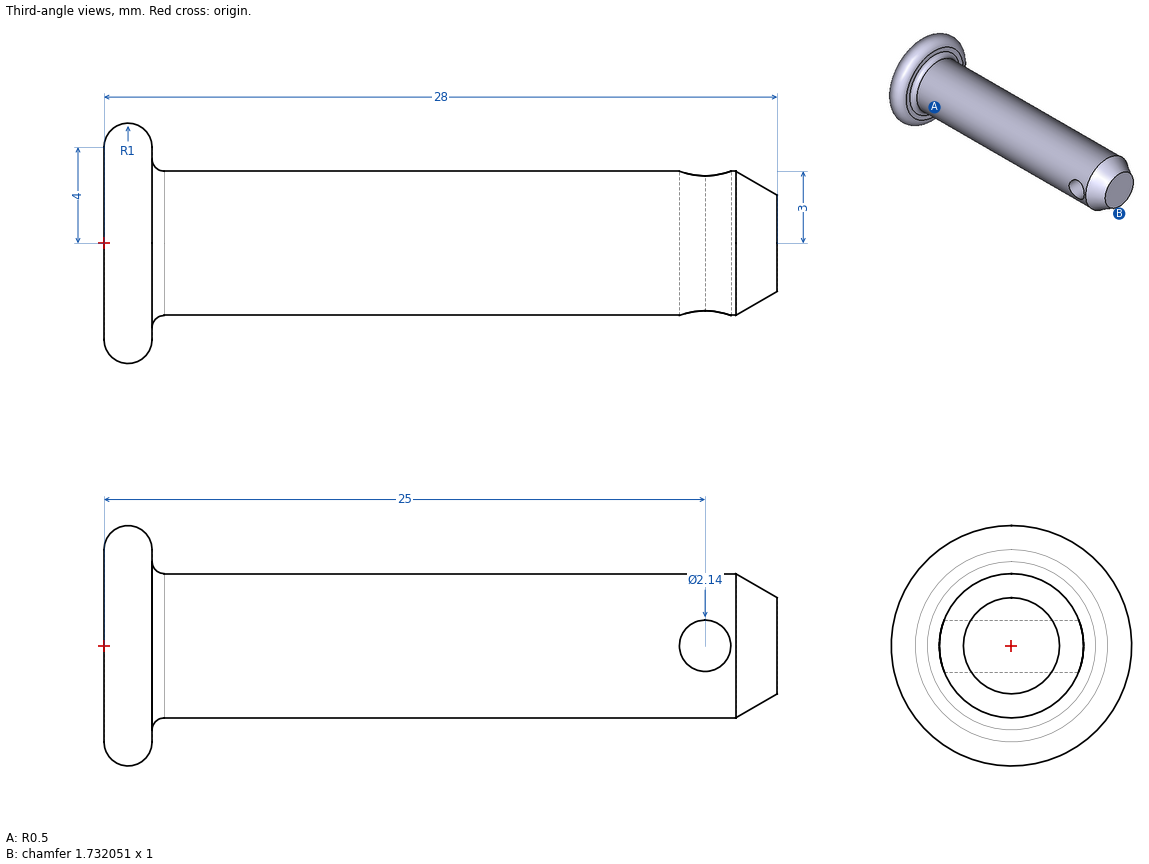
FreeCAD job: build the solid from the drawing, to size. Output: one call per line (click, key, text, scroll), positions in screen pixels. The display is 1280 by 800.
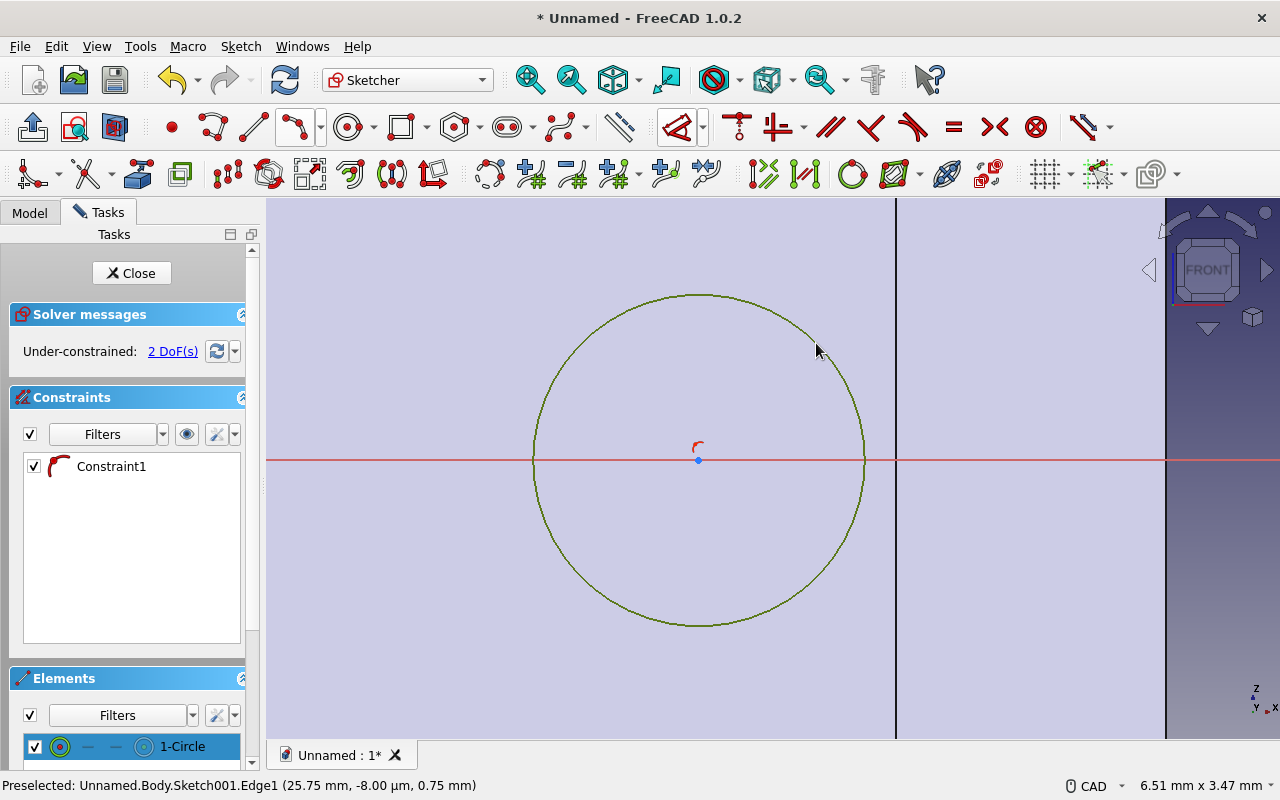
click(702, 128)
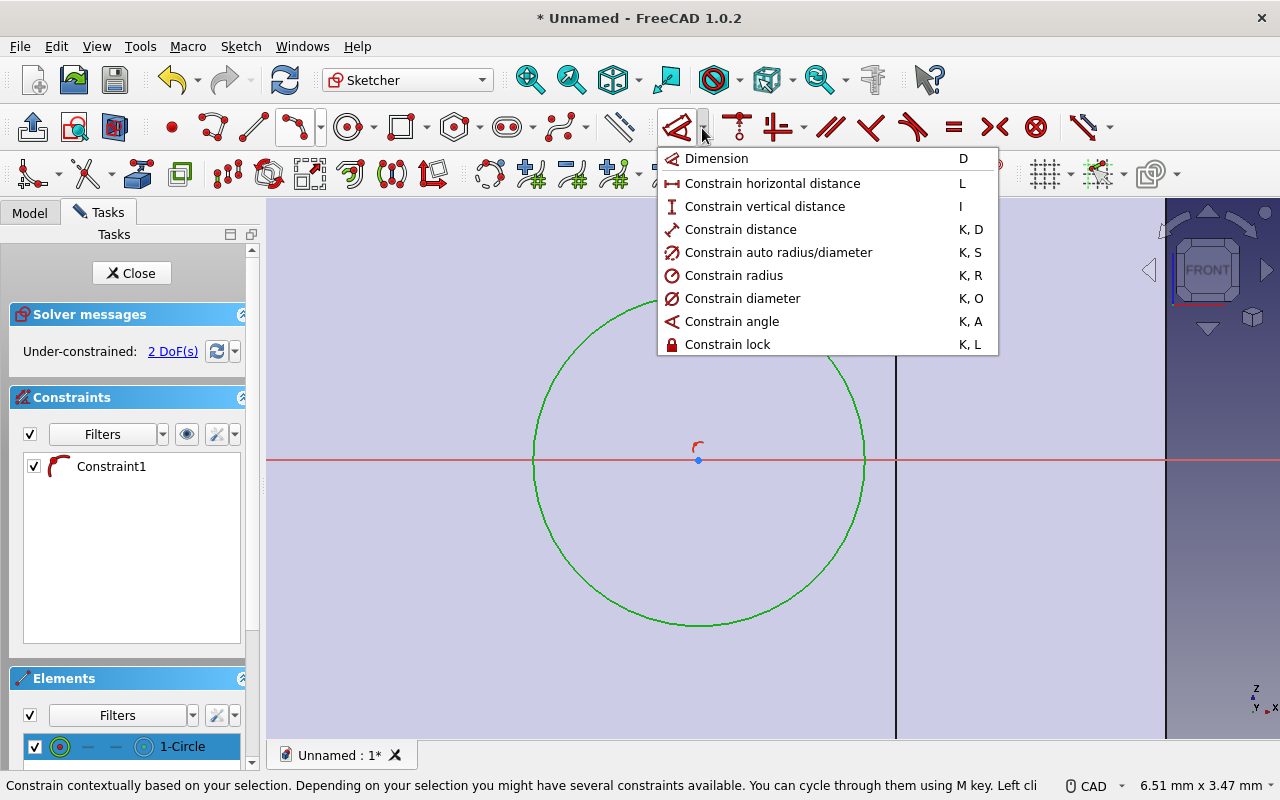
click(828, 298)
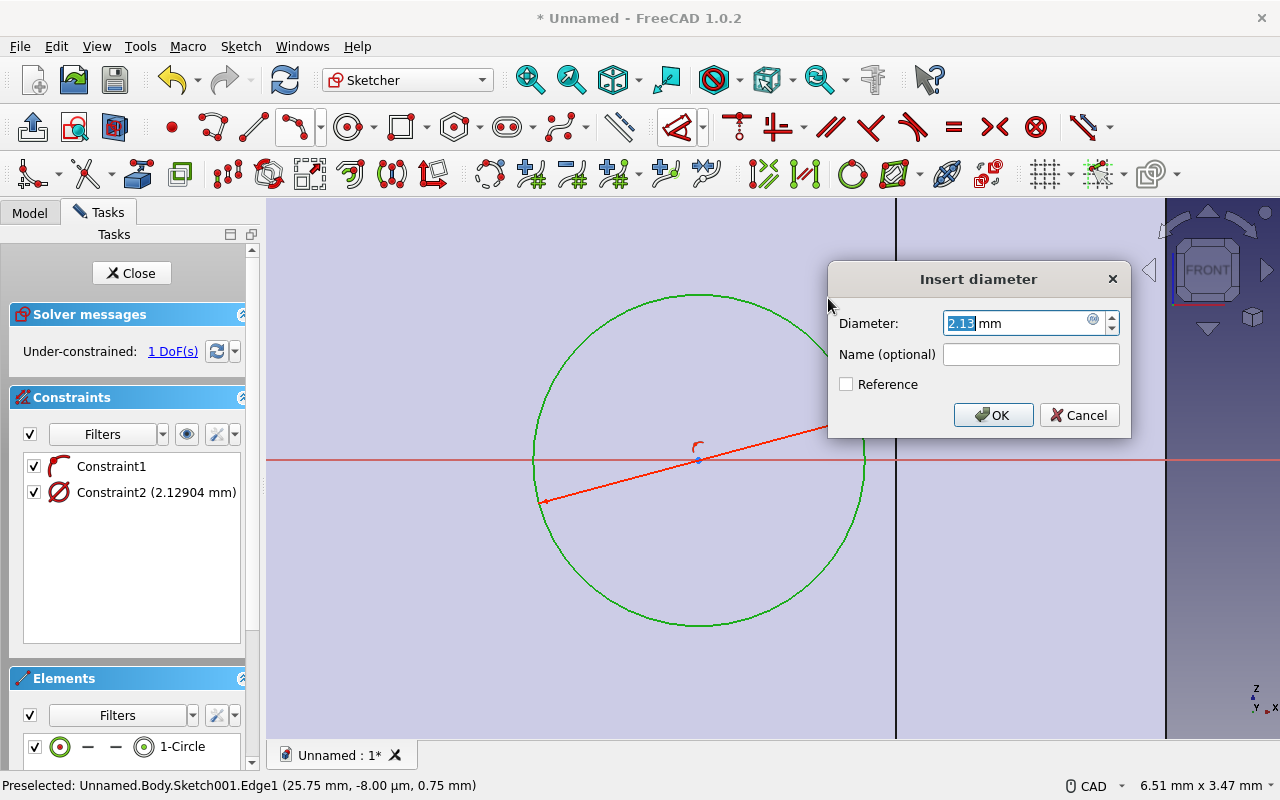
text(2.14)
key(Return)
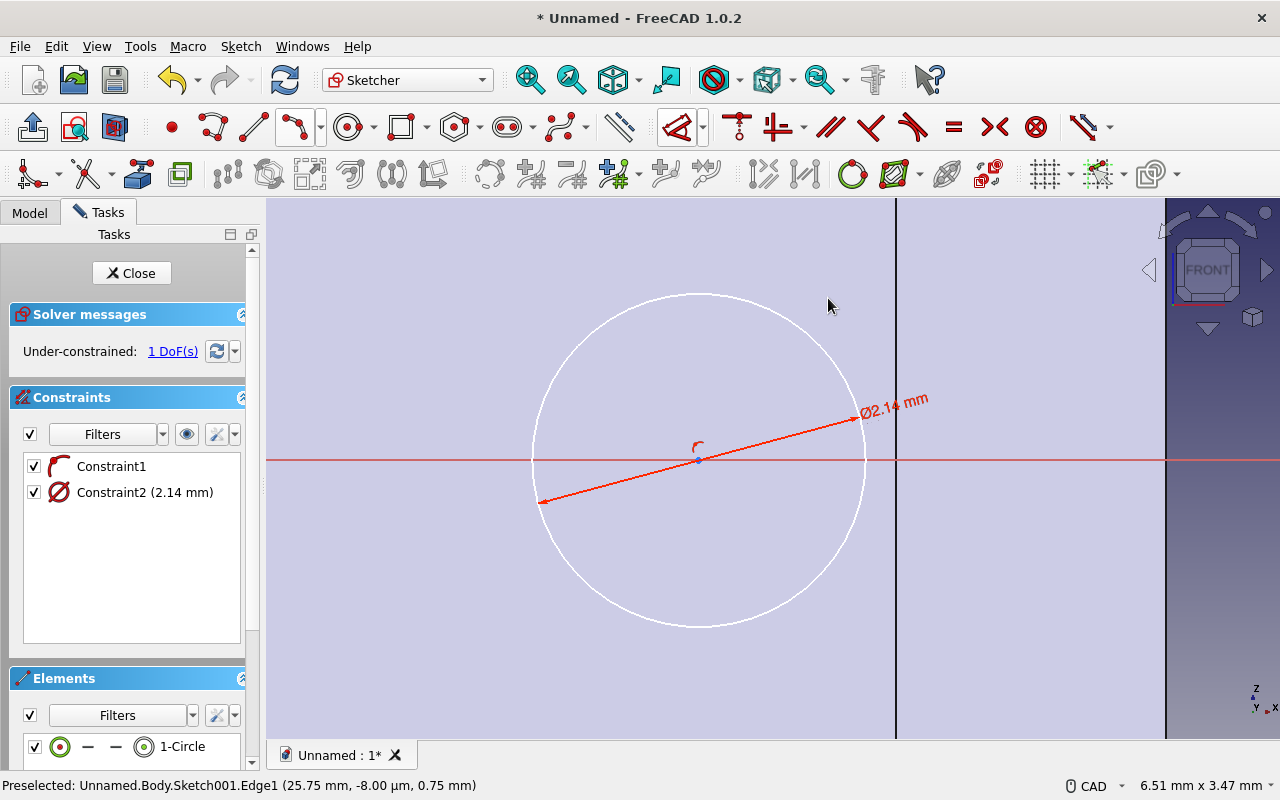
click(699, 460)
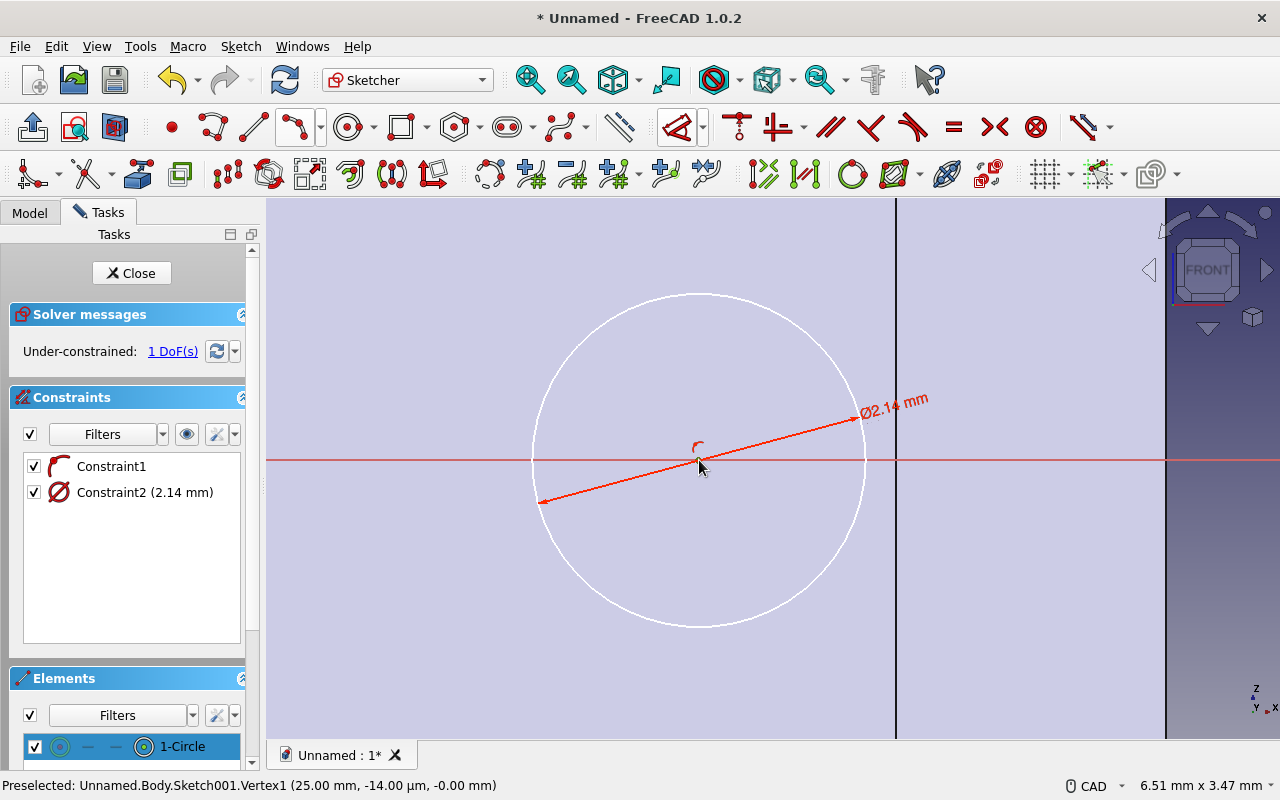
click(702, 128)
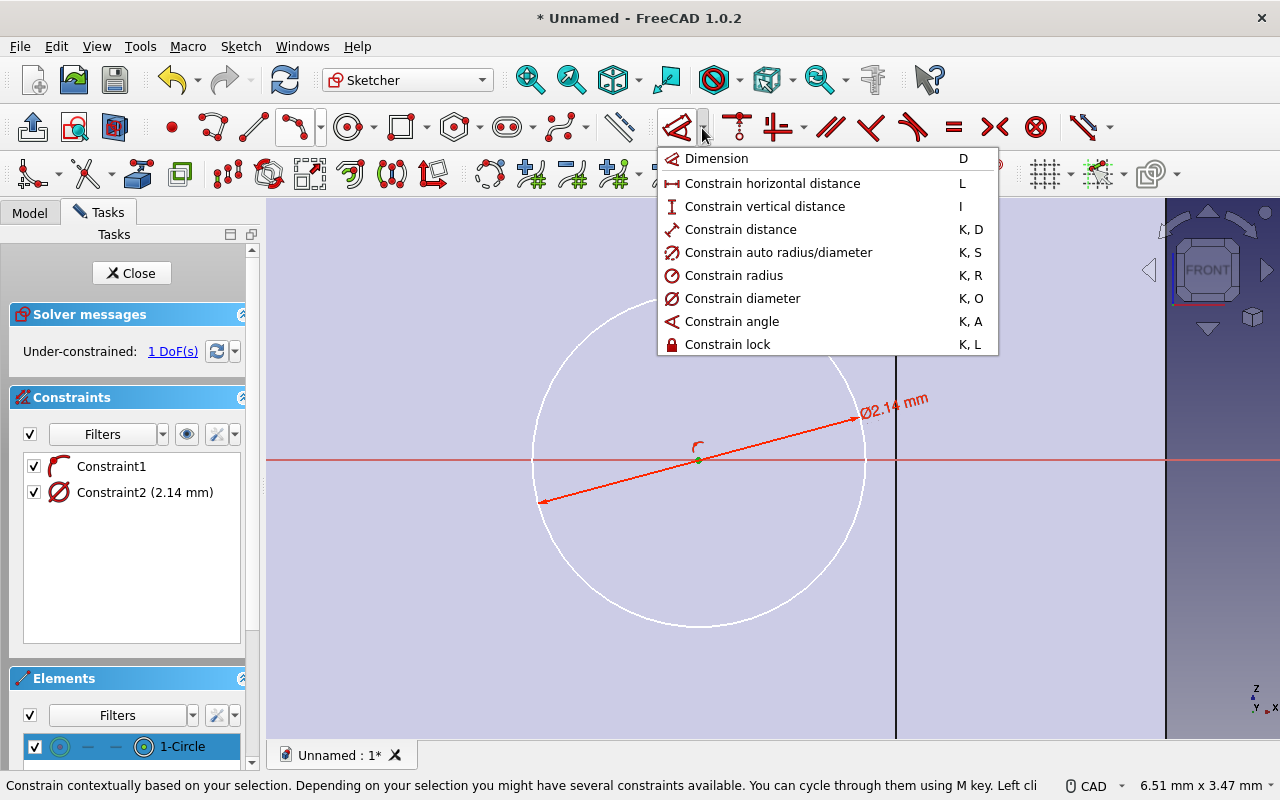
click(828, 184)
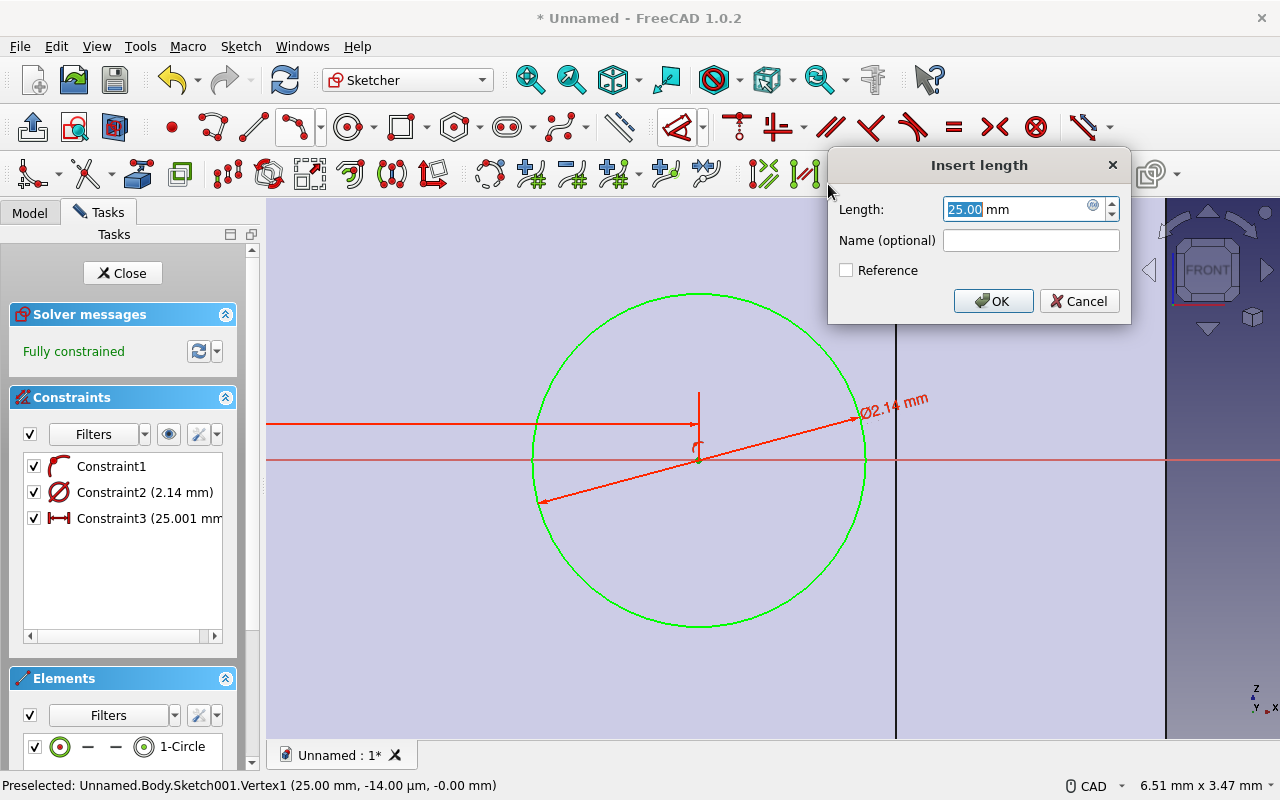
text(25)
key(Return)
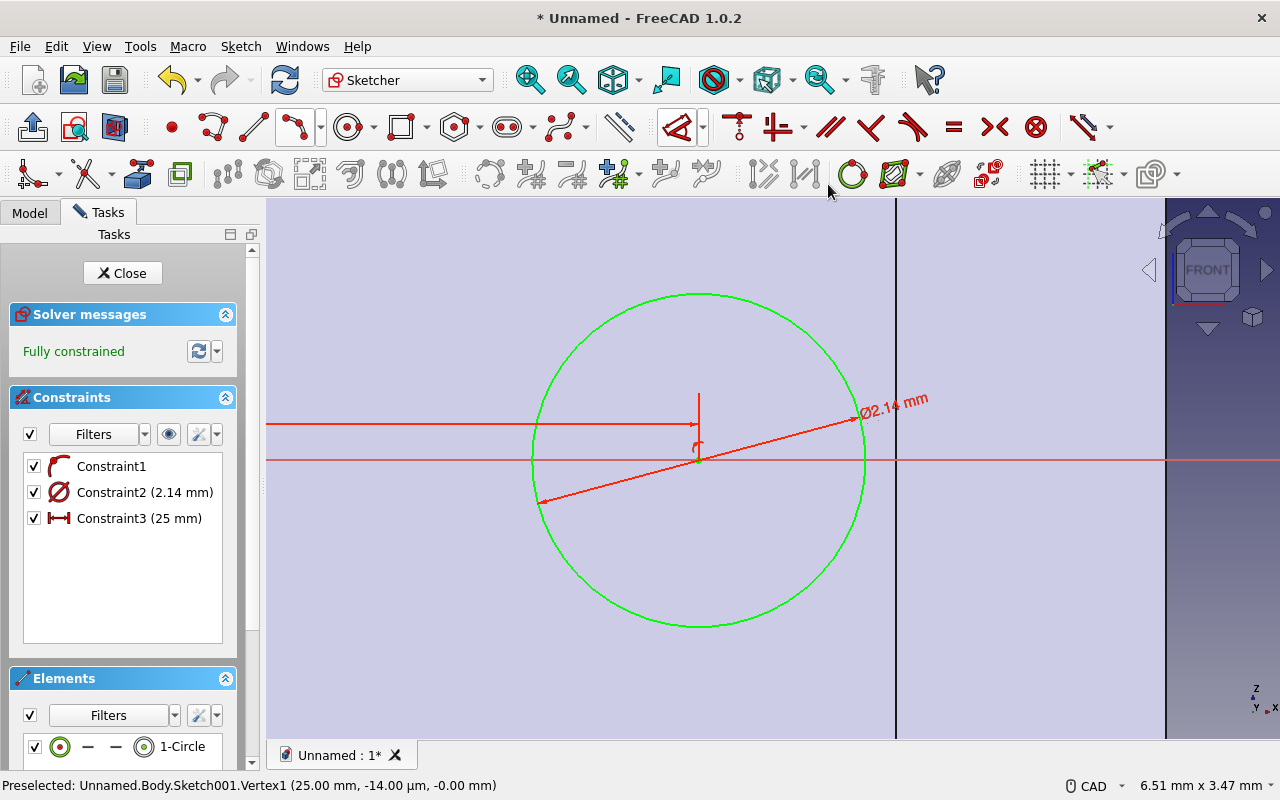
click(123, 273)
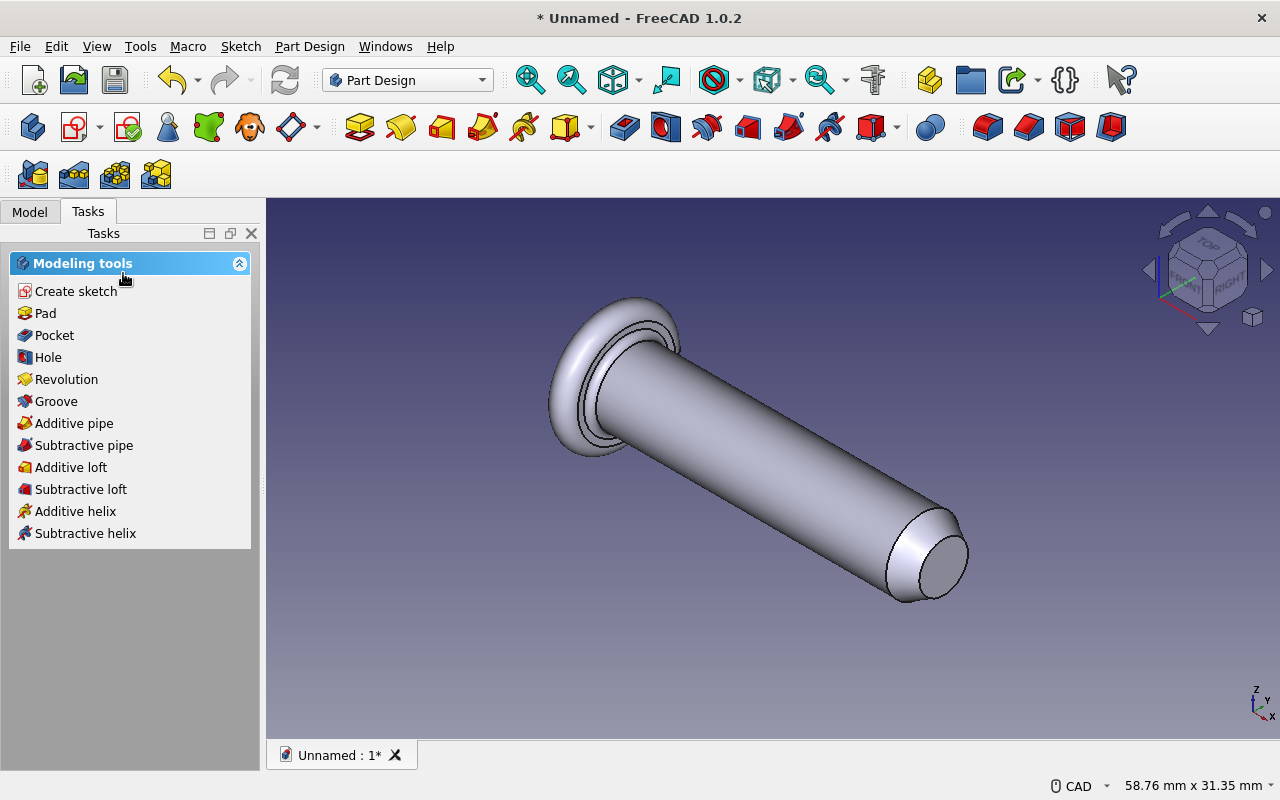
click(625, 128)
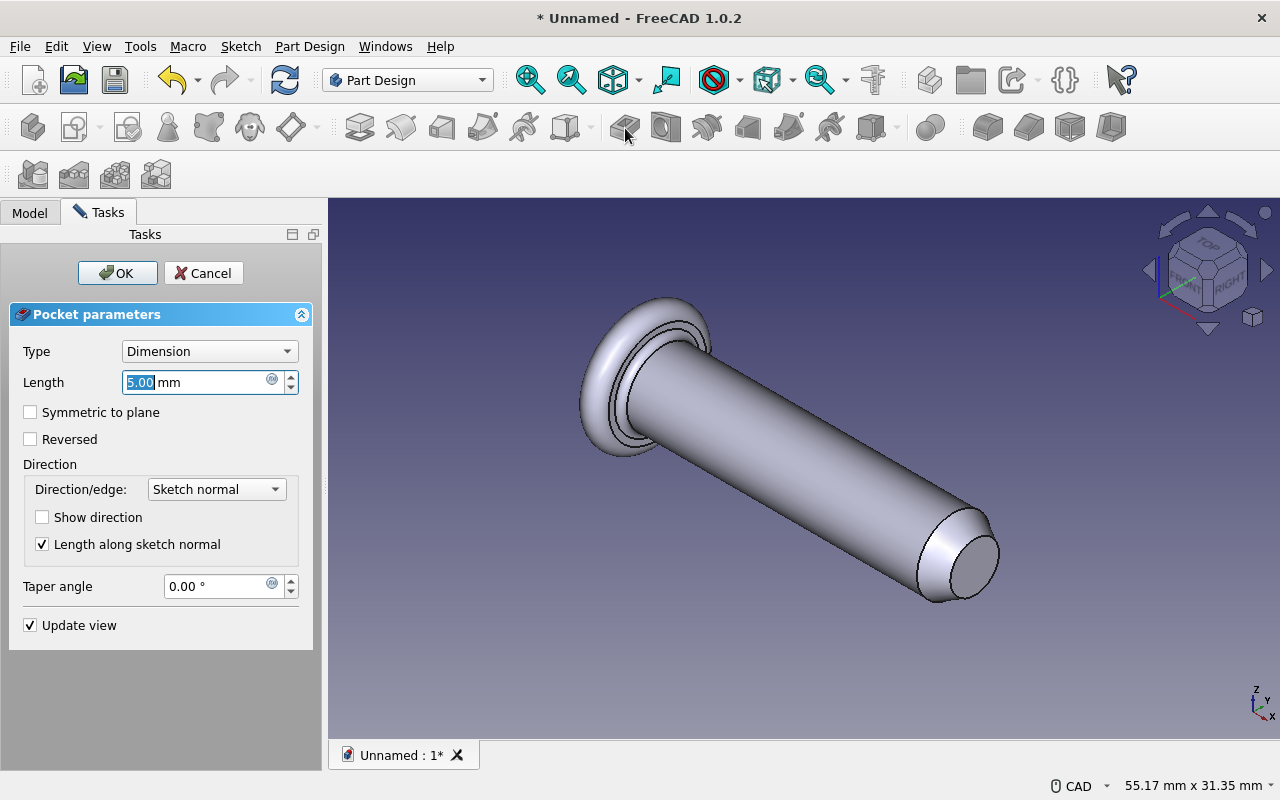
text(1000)
key(Tab)